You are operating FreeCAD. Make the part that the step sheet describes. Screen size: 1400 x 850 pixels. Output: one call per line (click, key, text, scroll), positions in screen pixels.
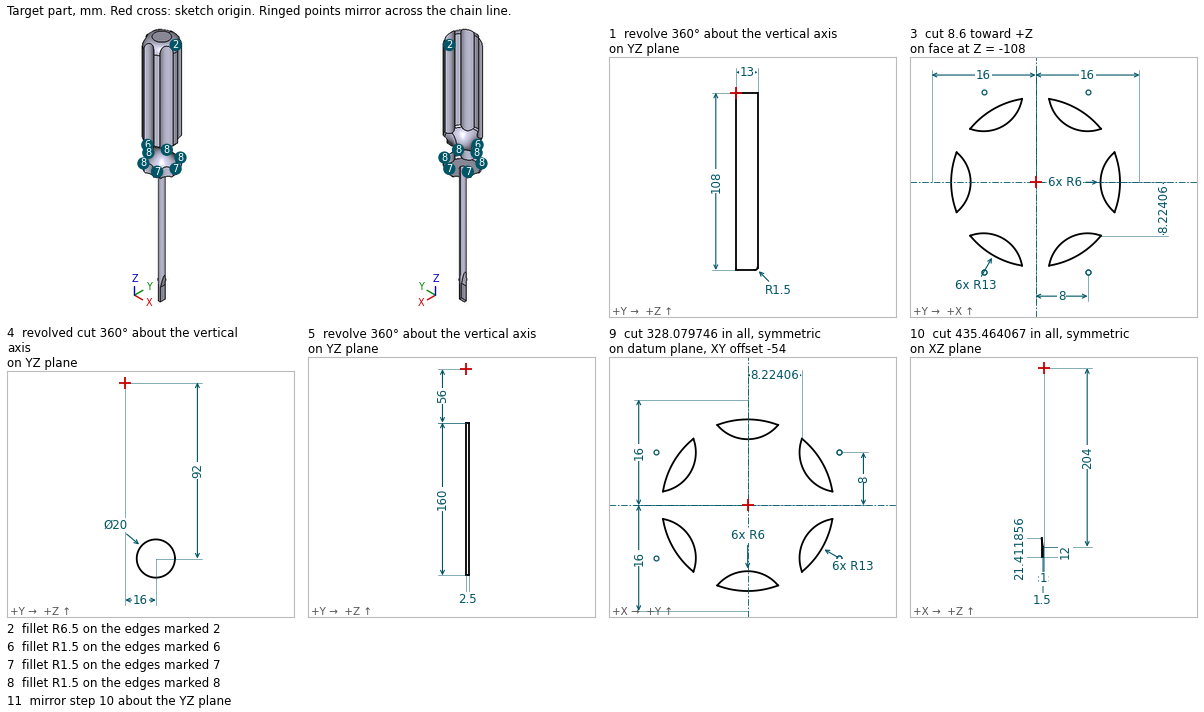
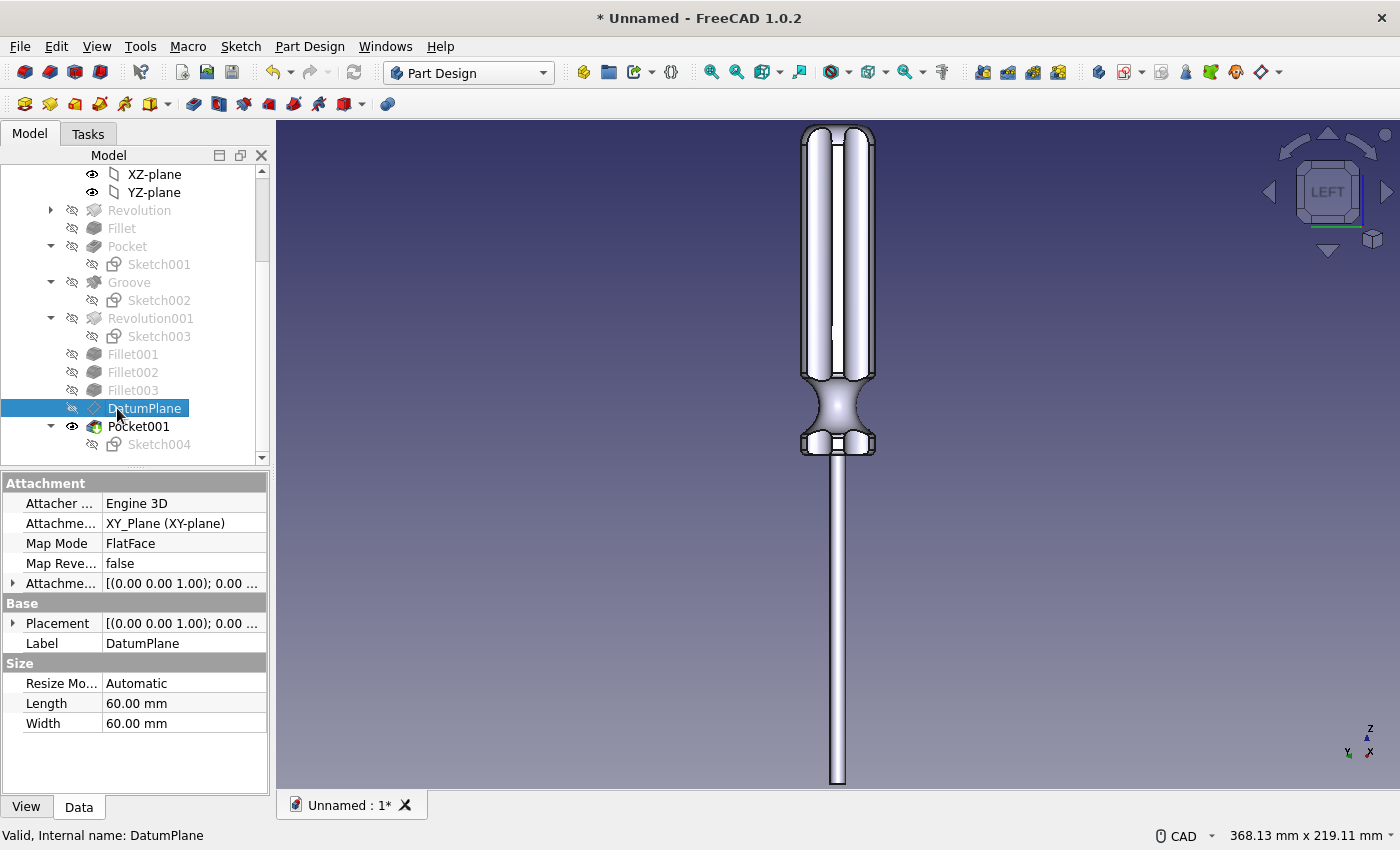
click(316, 749)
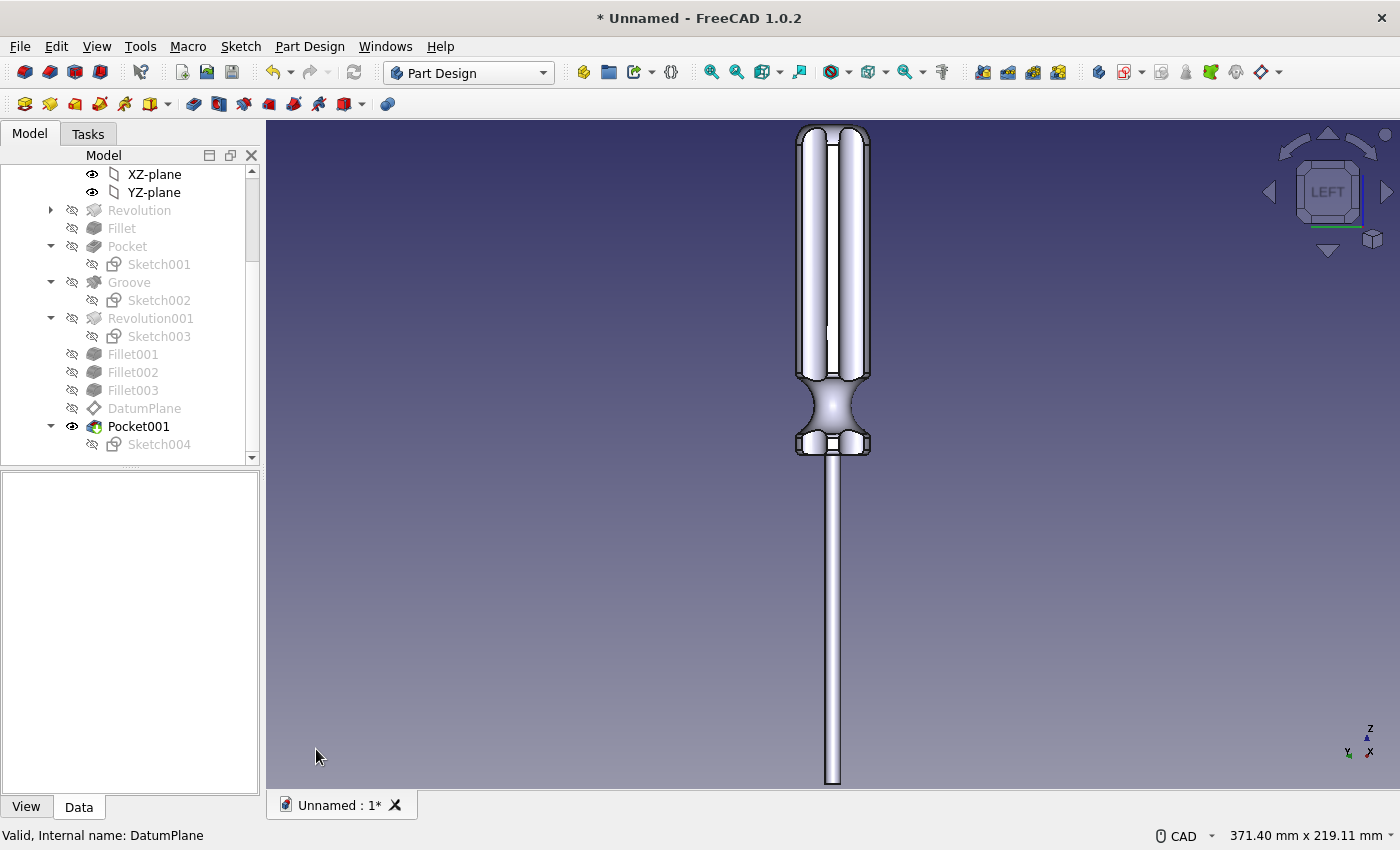
click(1124, 72)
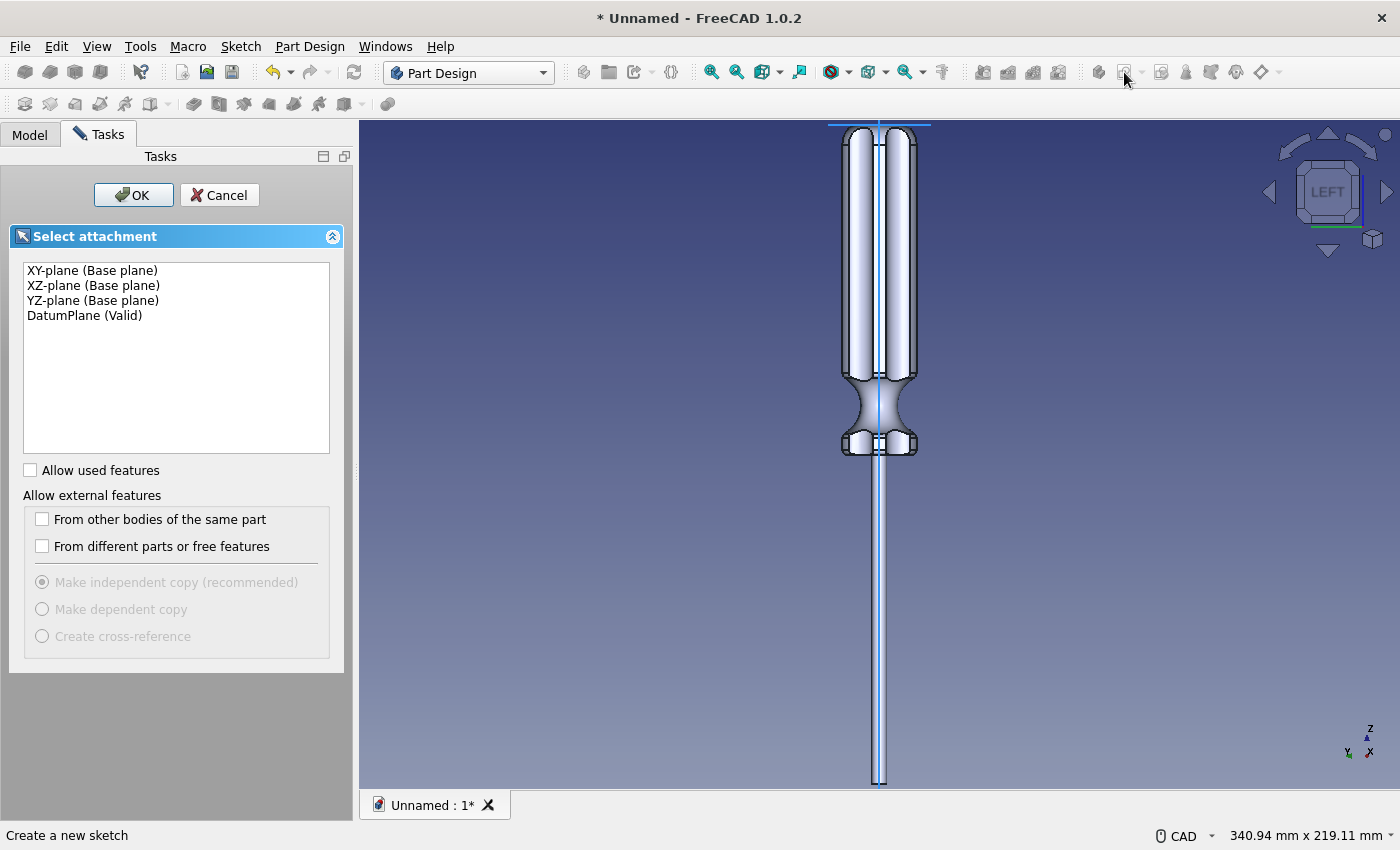
click(84, 286)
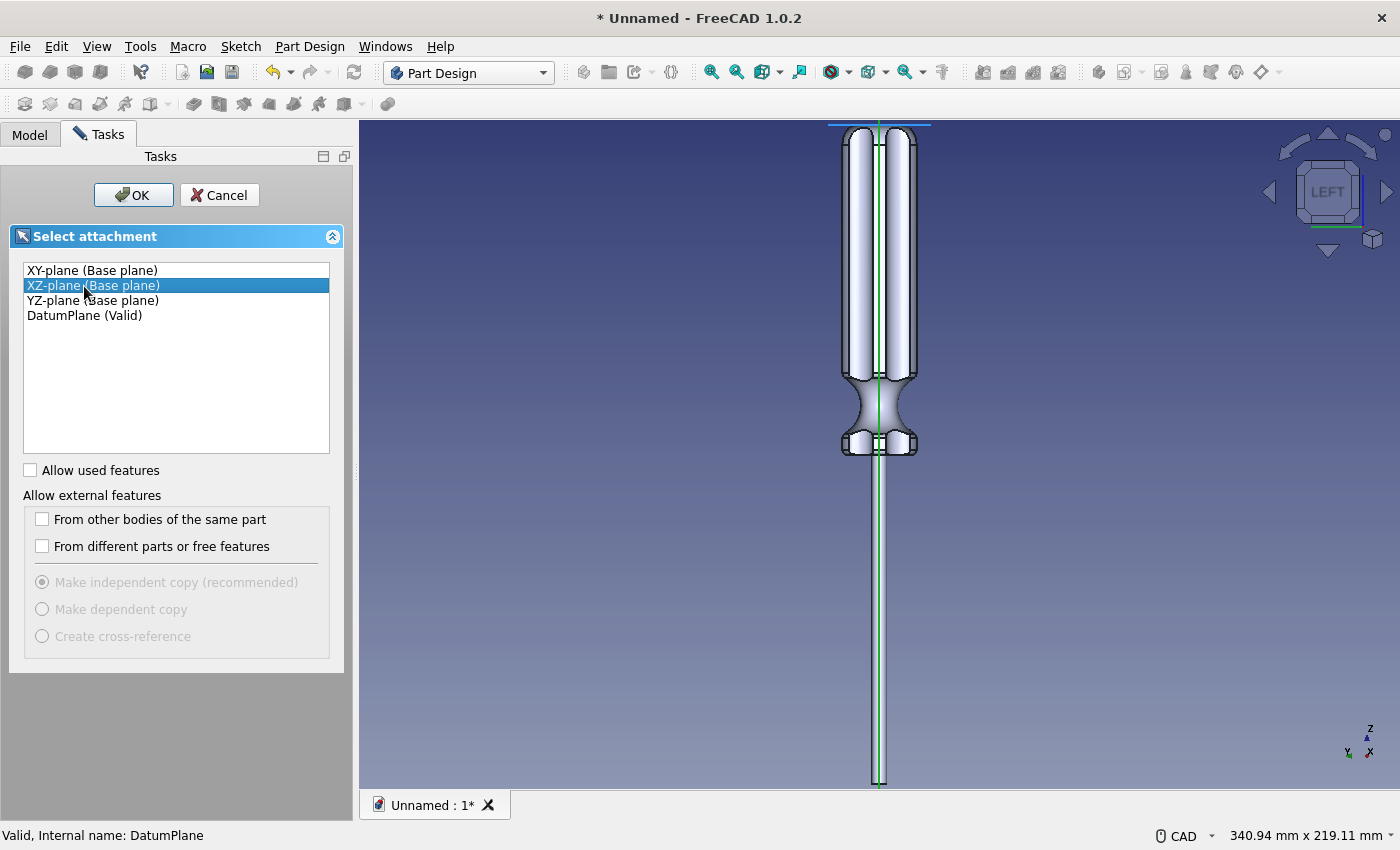
click(134, 195)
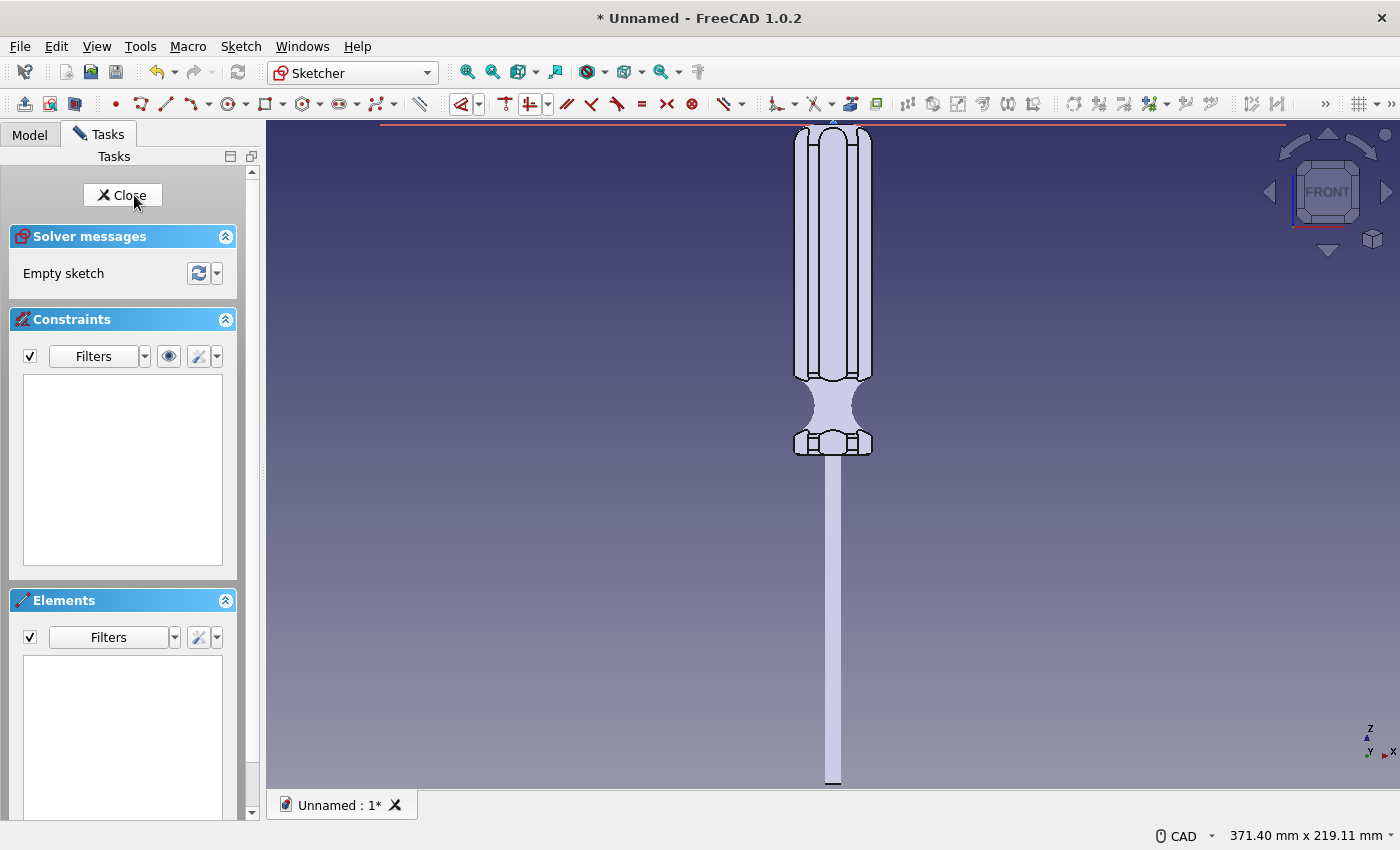
key(q)
key(s)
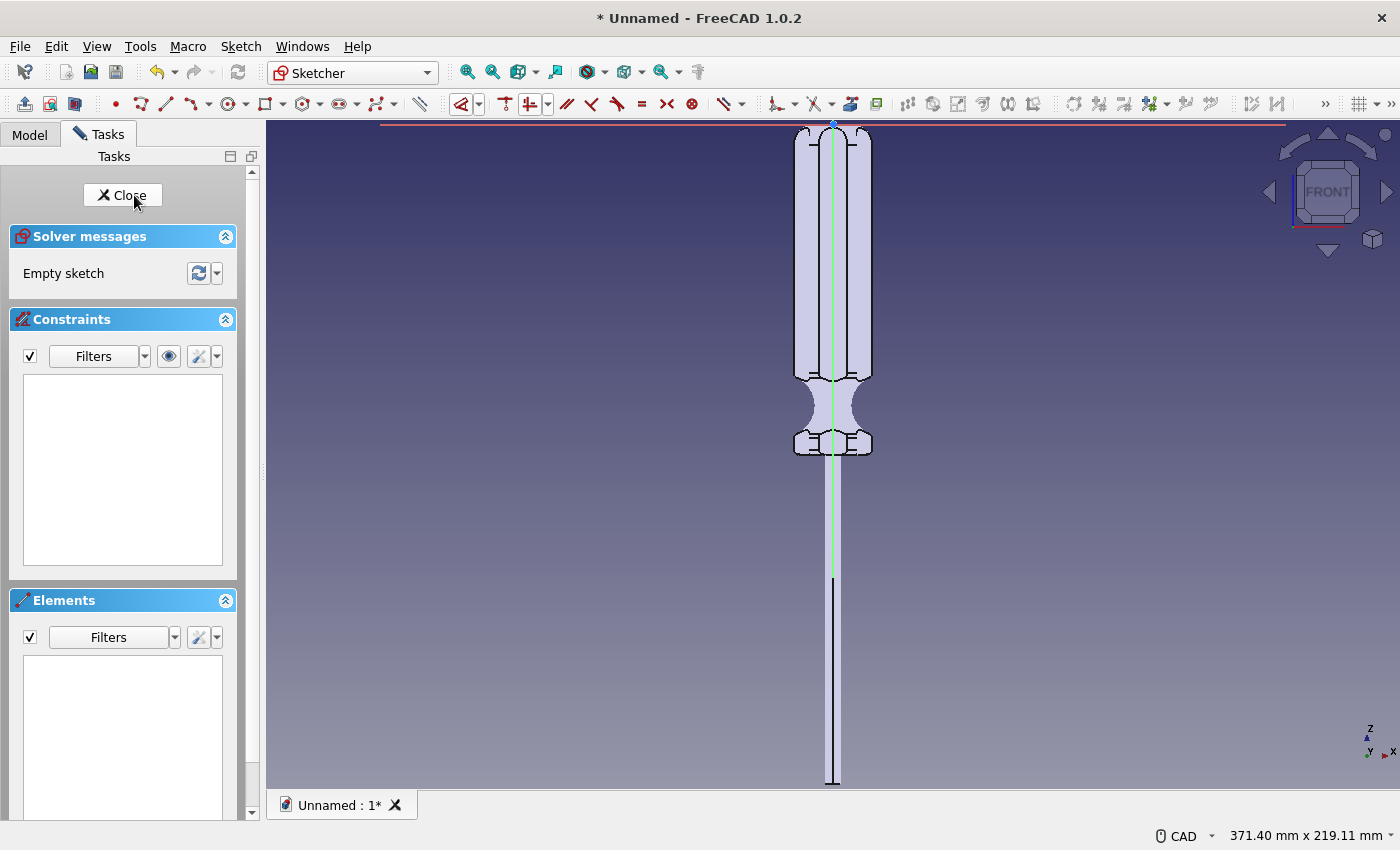
scroll(764, 454, down, 5)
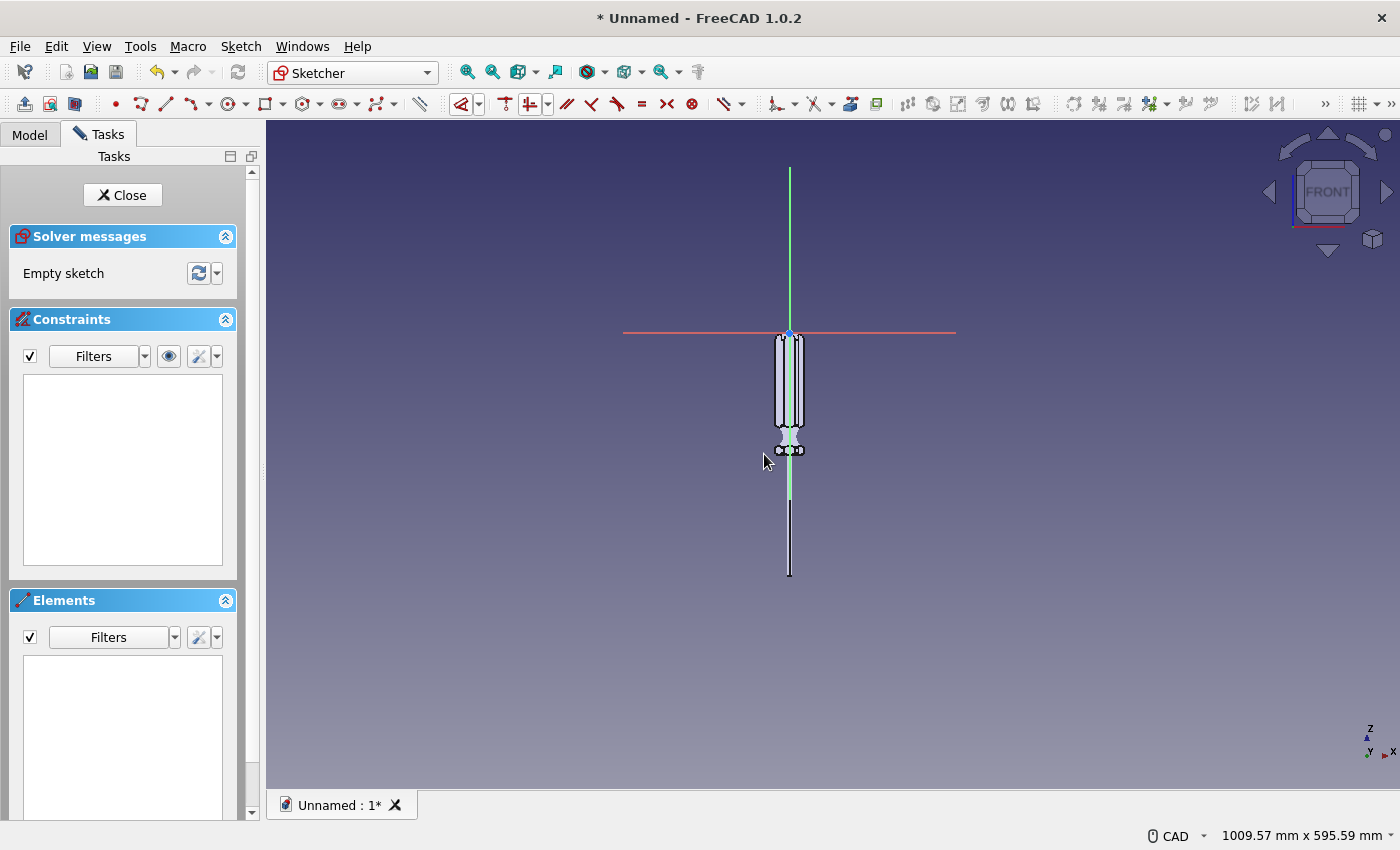
scroll(789, 571, up, 14)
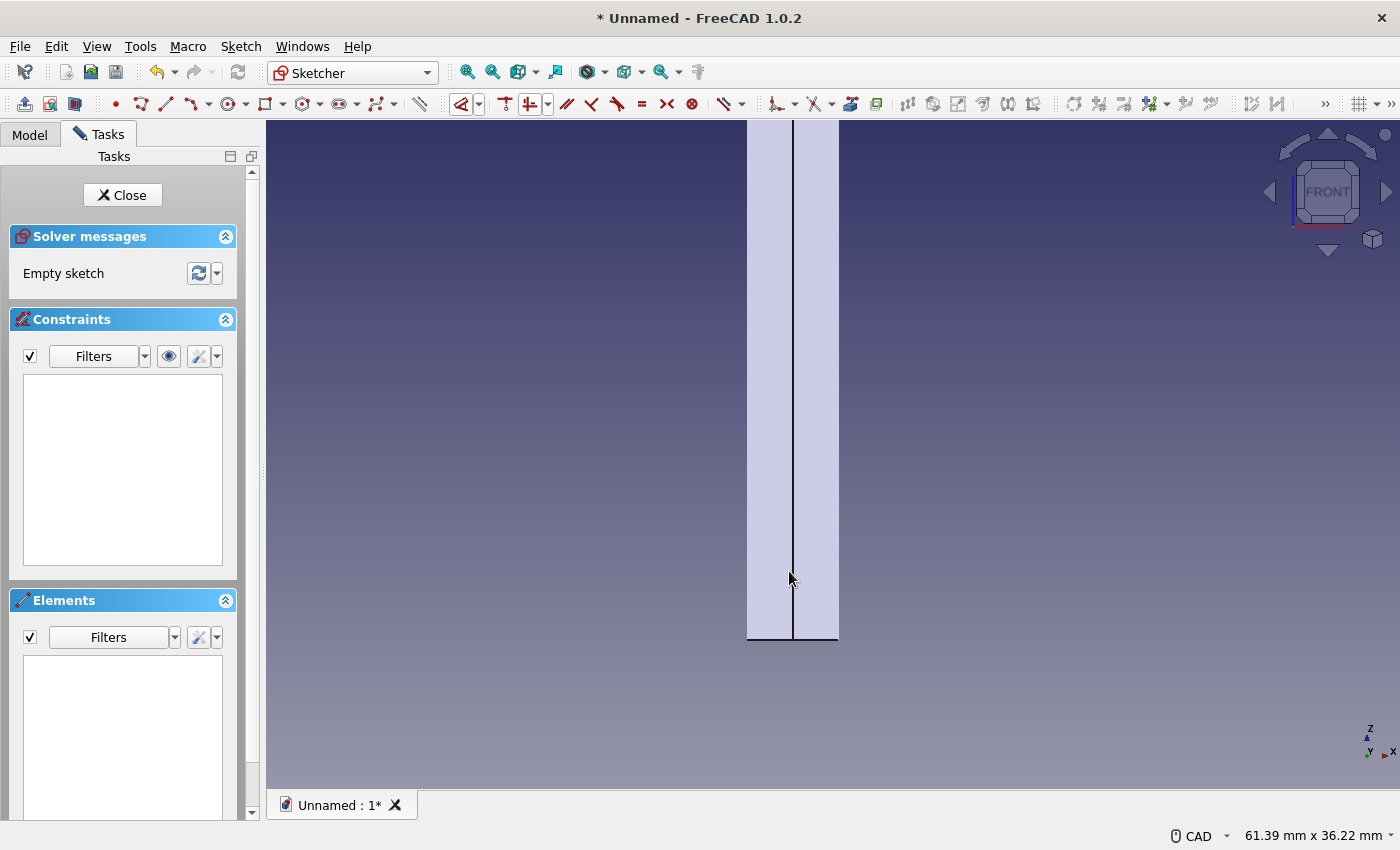
key(g)
key(m)